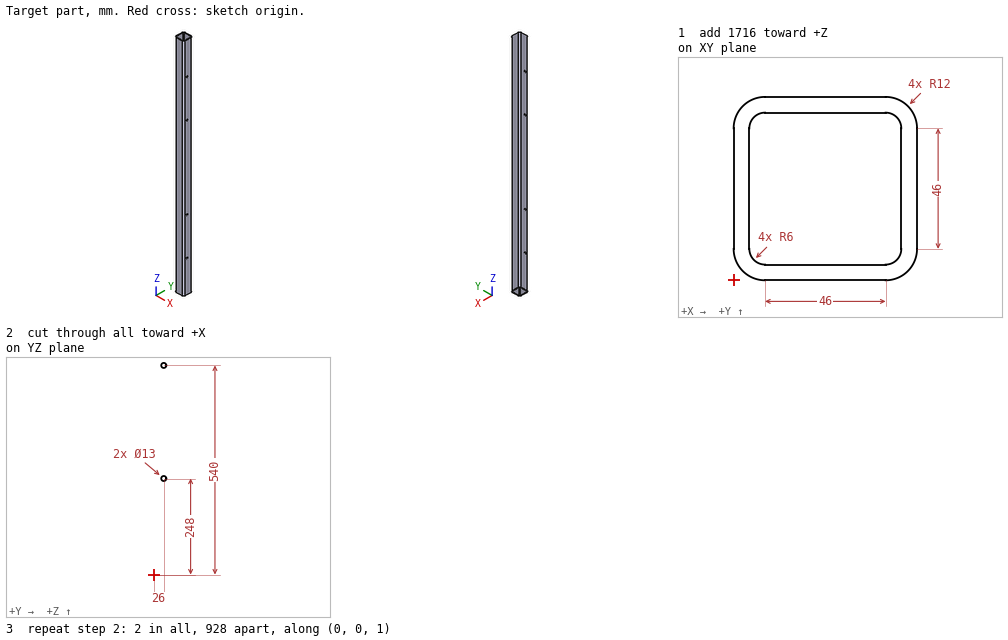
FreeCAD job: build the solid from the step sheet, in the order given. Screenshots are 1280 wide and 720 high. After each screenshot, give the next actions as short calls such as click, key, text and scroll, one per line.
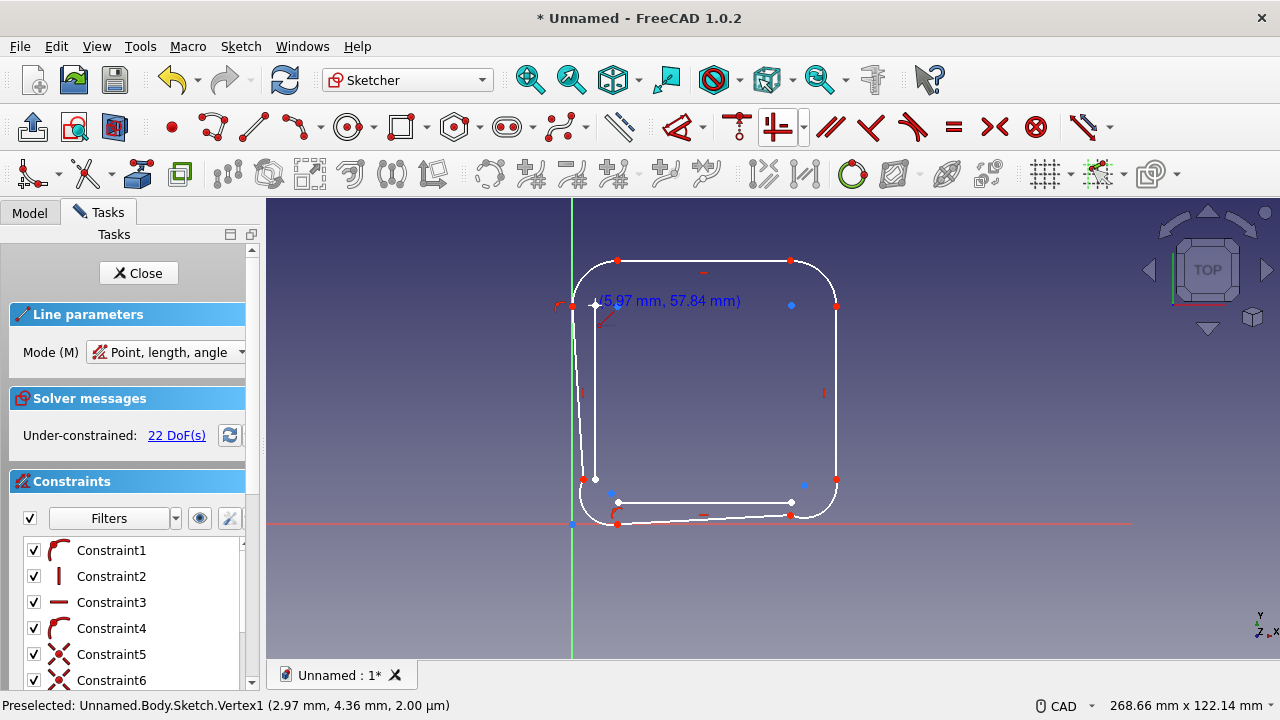
click(618, 283)
click(791, 283)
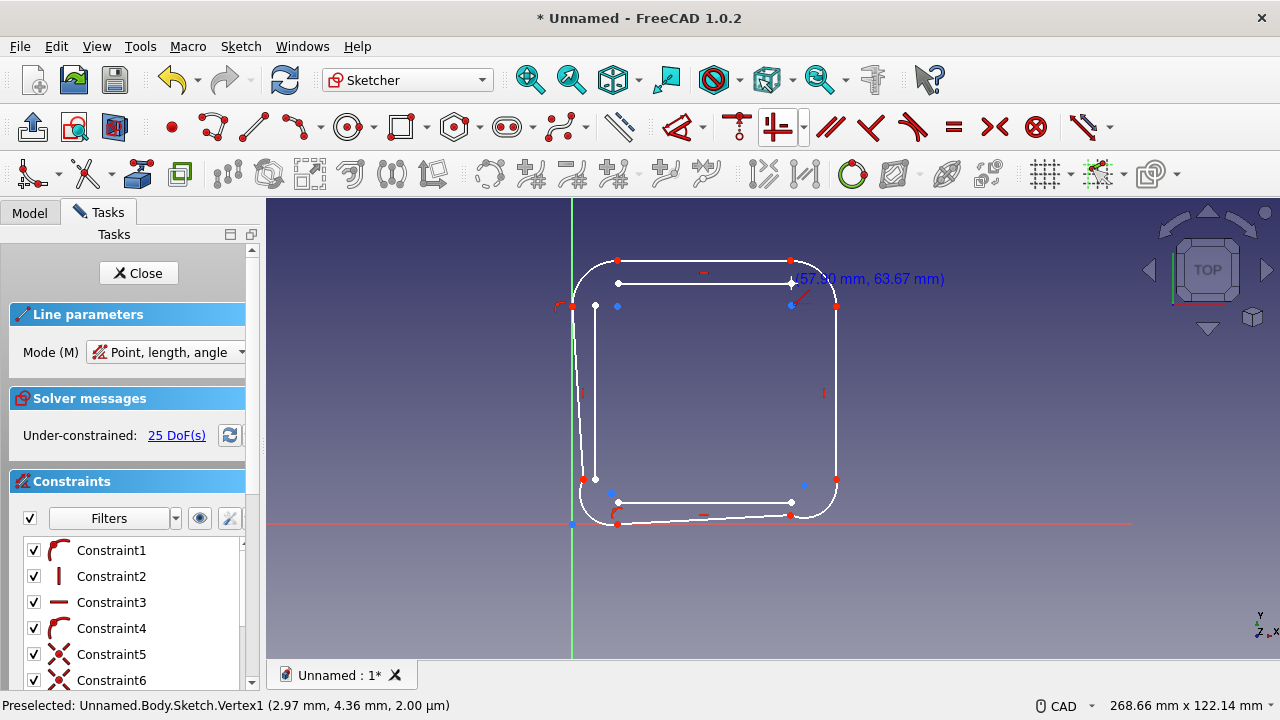
click(814, 305)
click(814, 479)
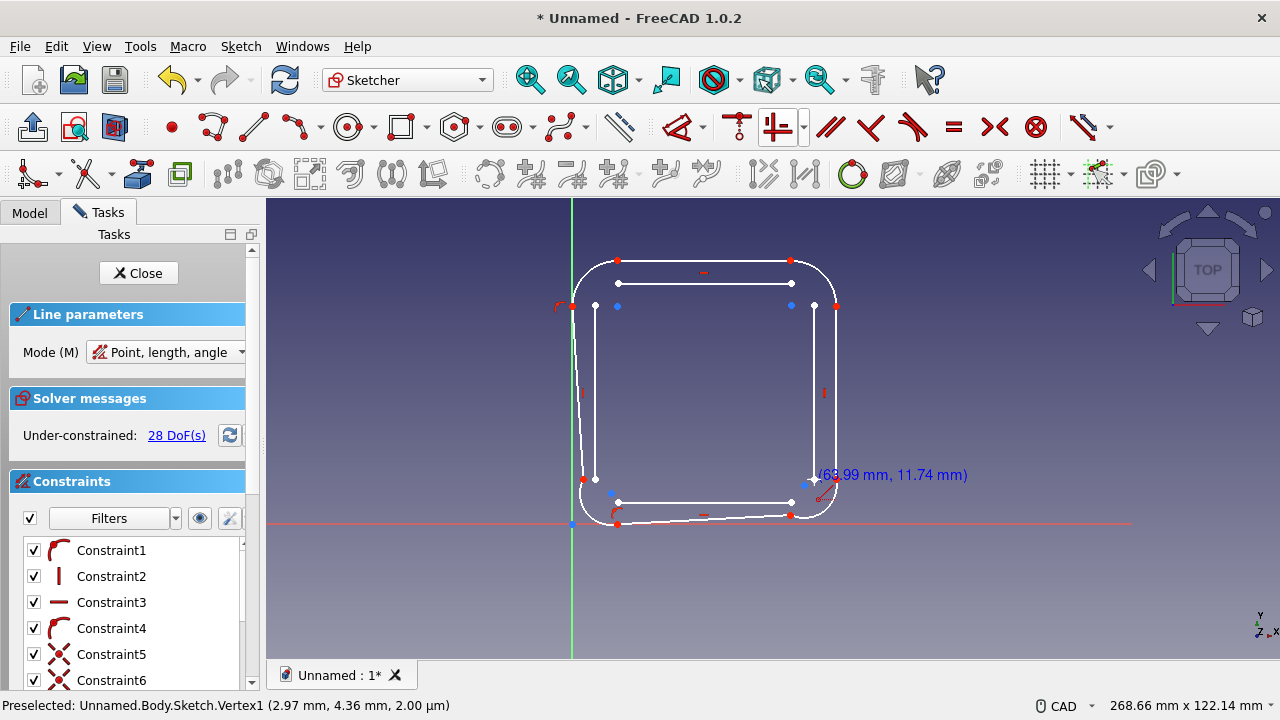
click(294, 128)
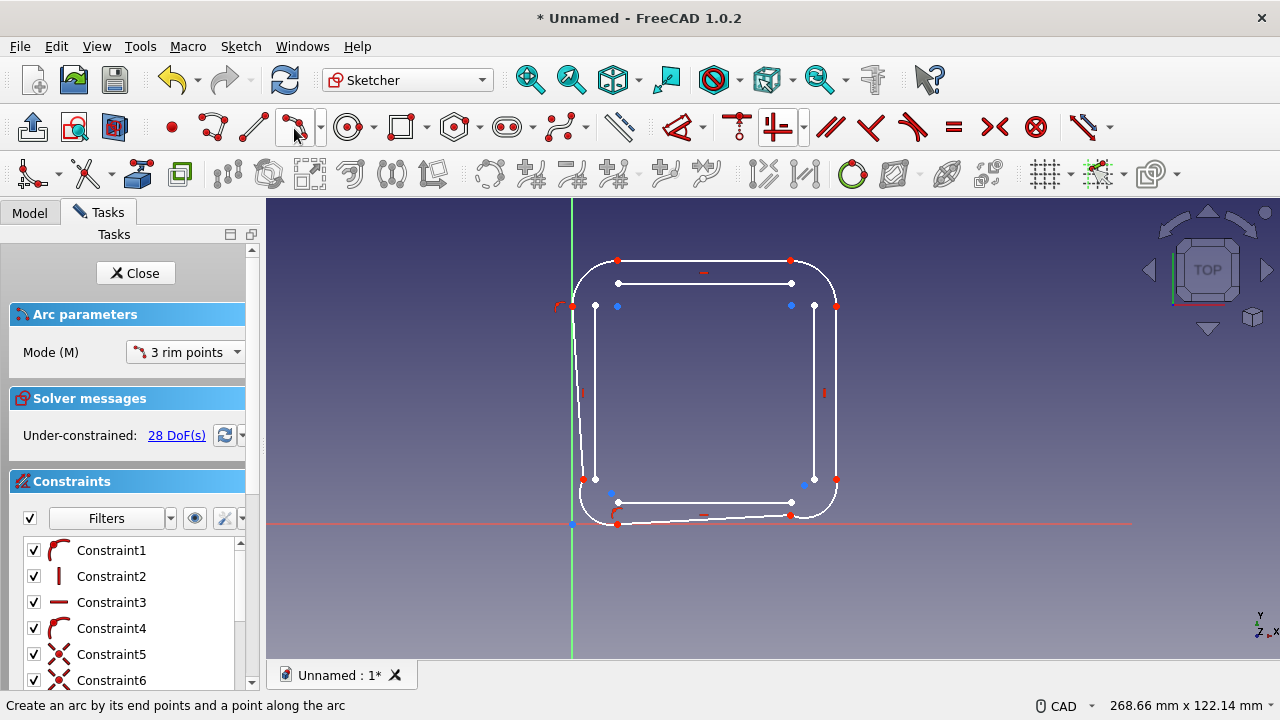
click(618, 503)
click(595, 480)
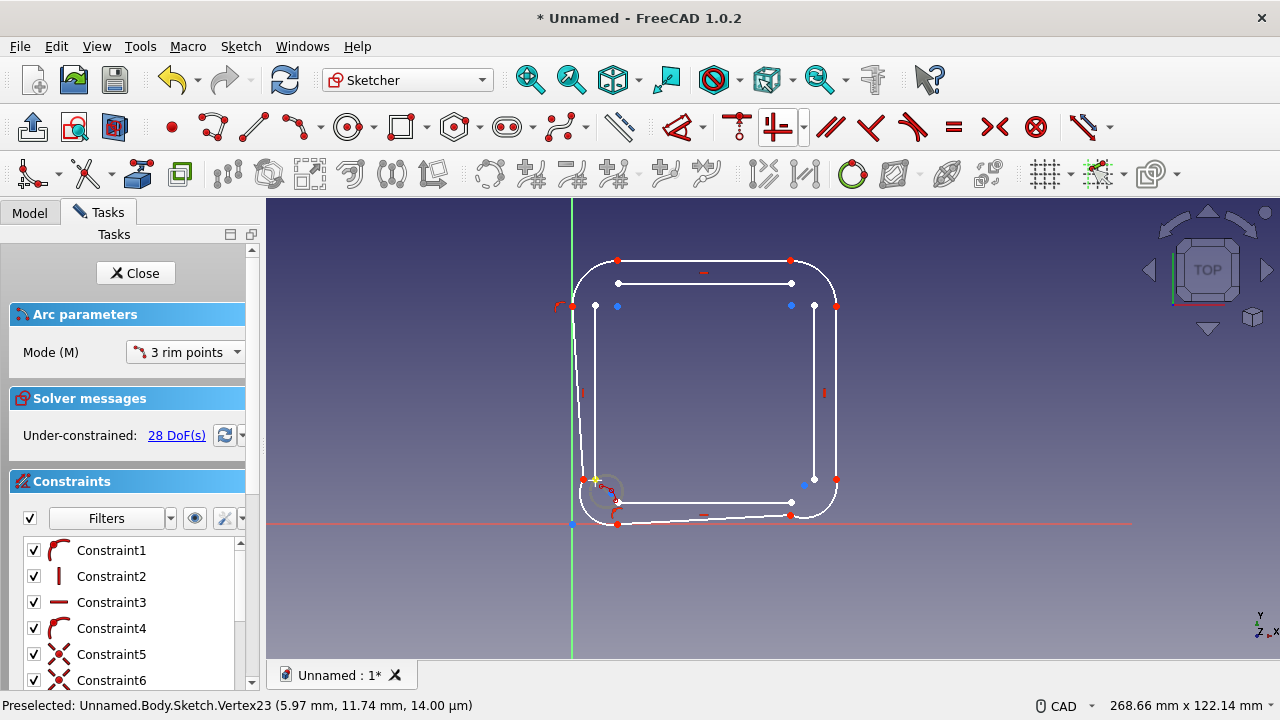
scroll(602, 495, up, 5)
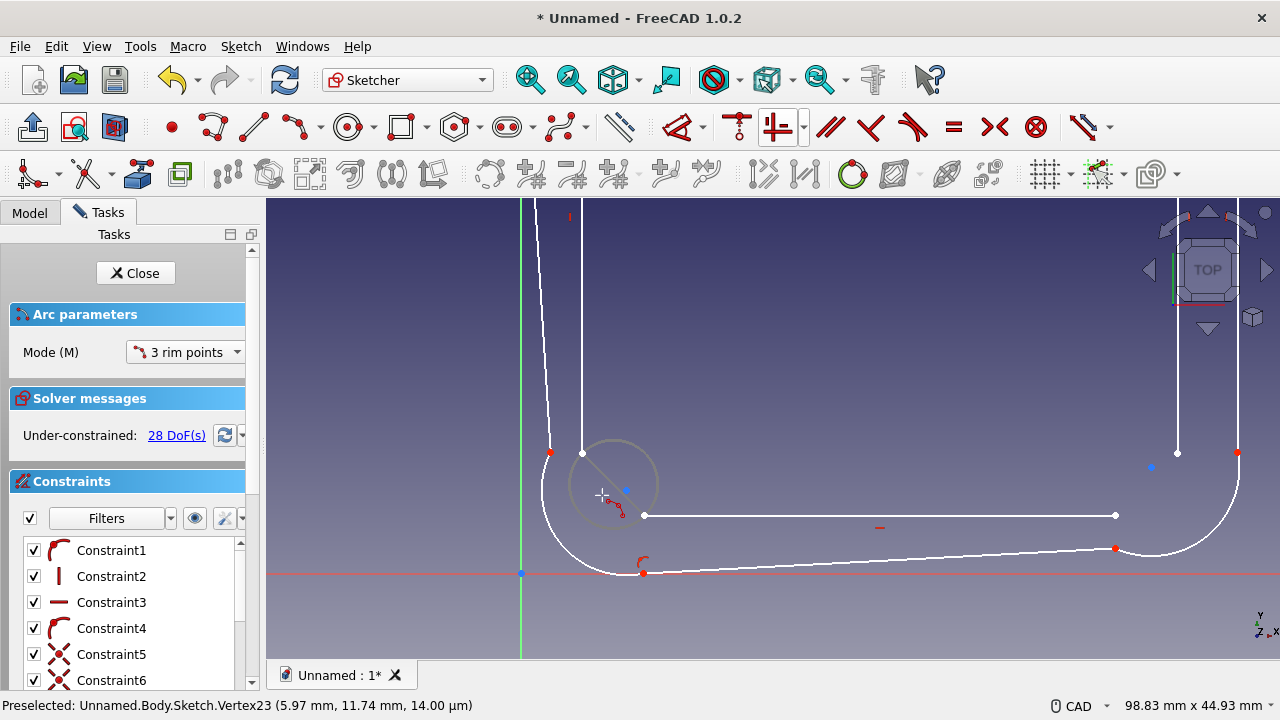
click(601, 494)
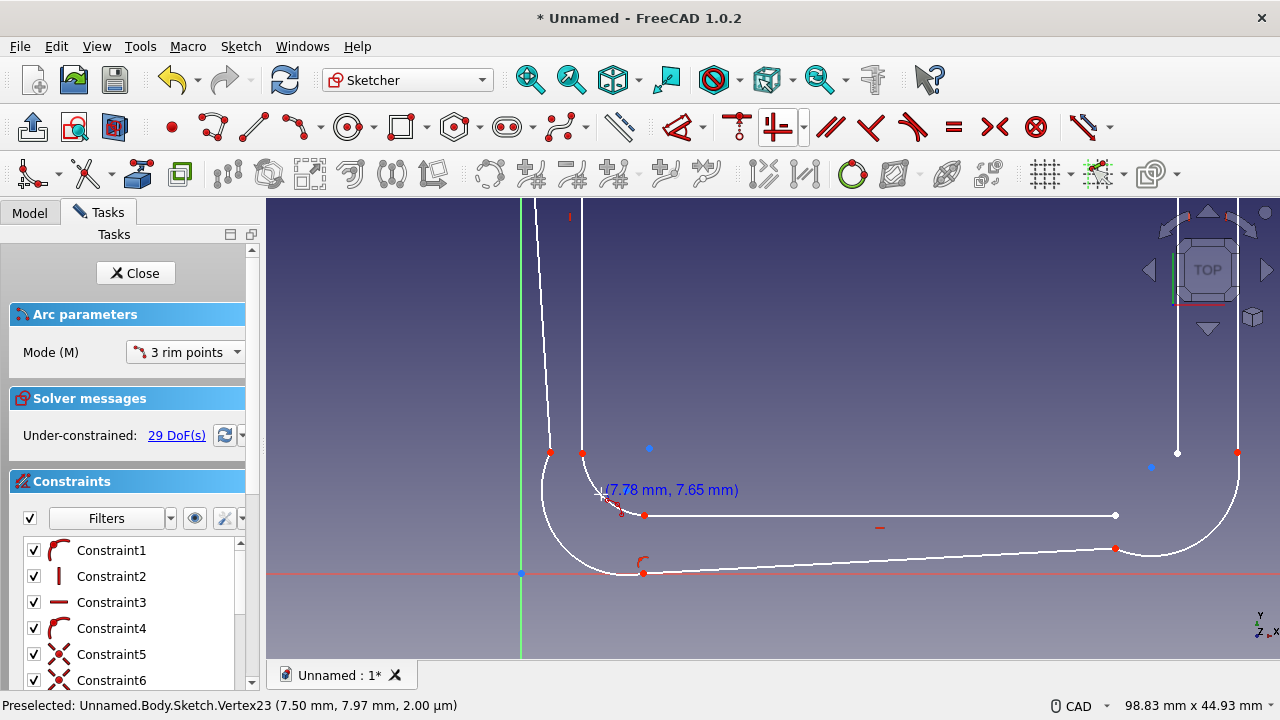
scroll(602, 553, down, 5)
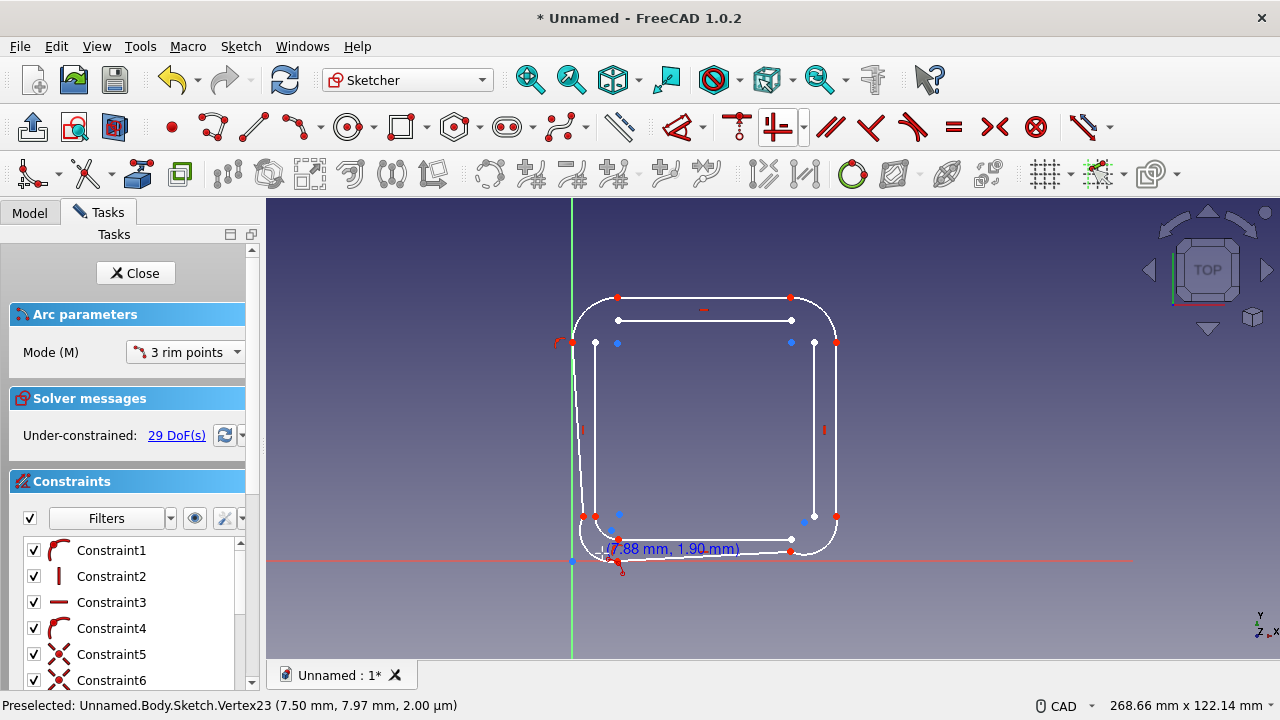
click(595, 343)
click(618, 321)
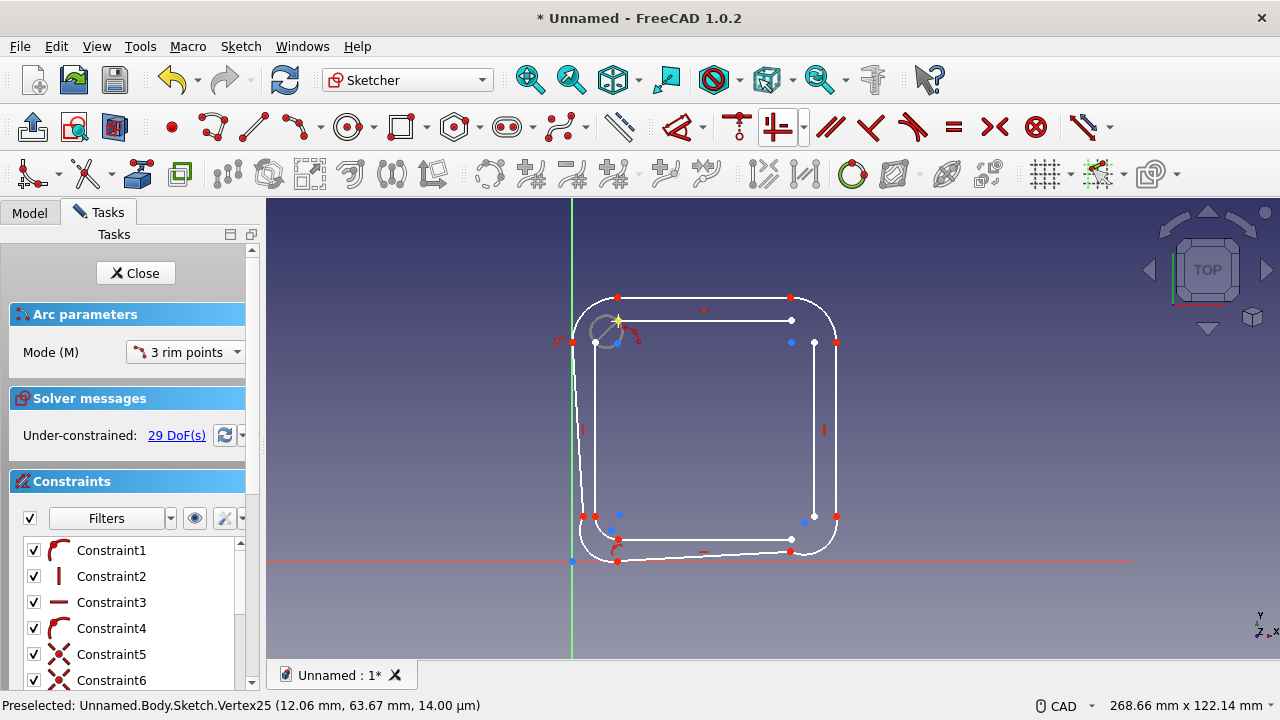
scroll(602, 326, up, 5)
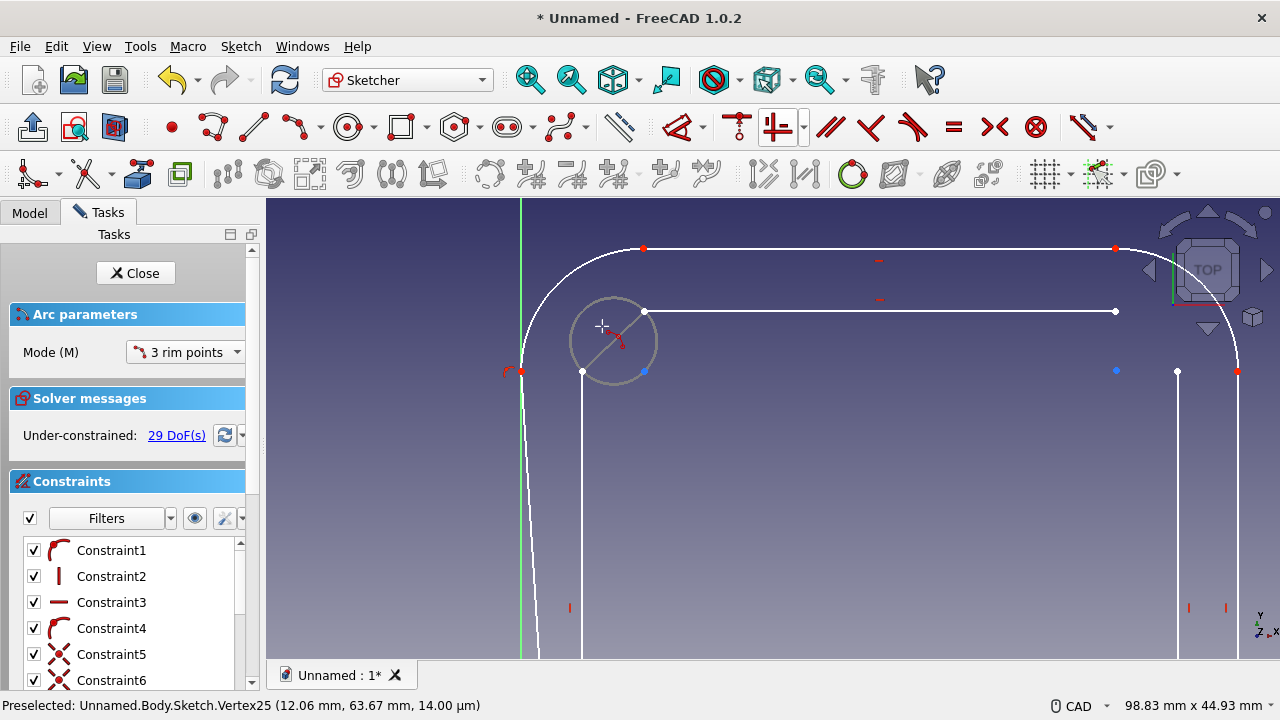
click(601, 326)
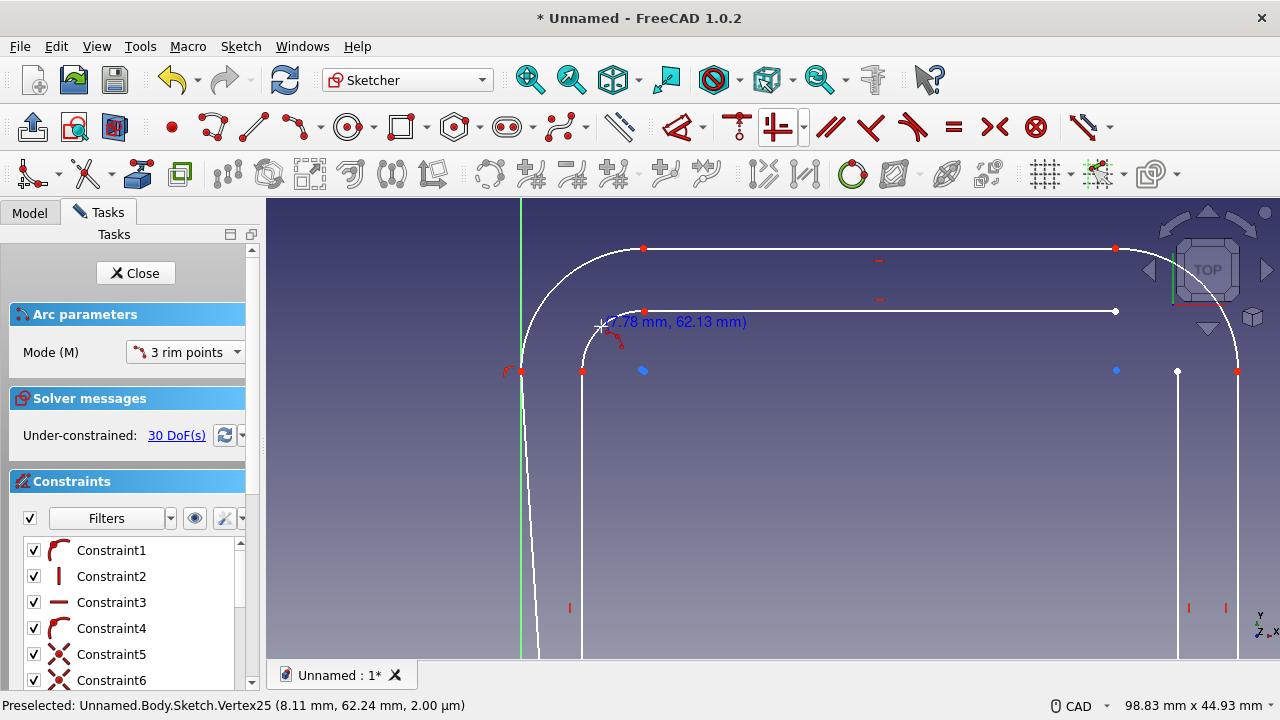
scroll(602, 326, down, 5)